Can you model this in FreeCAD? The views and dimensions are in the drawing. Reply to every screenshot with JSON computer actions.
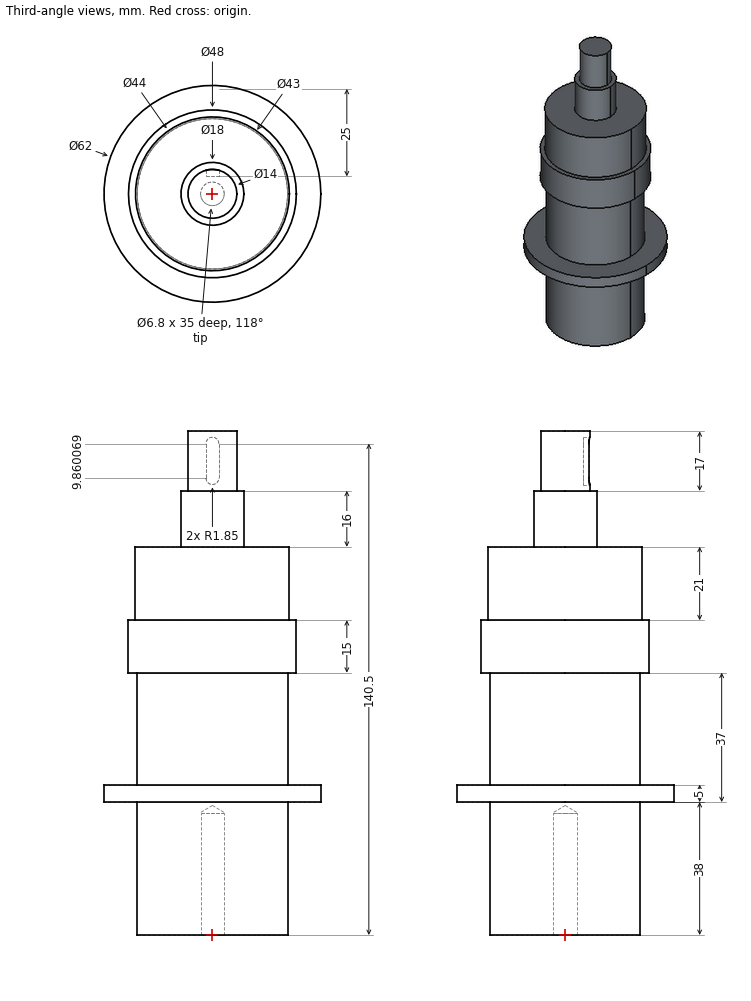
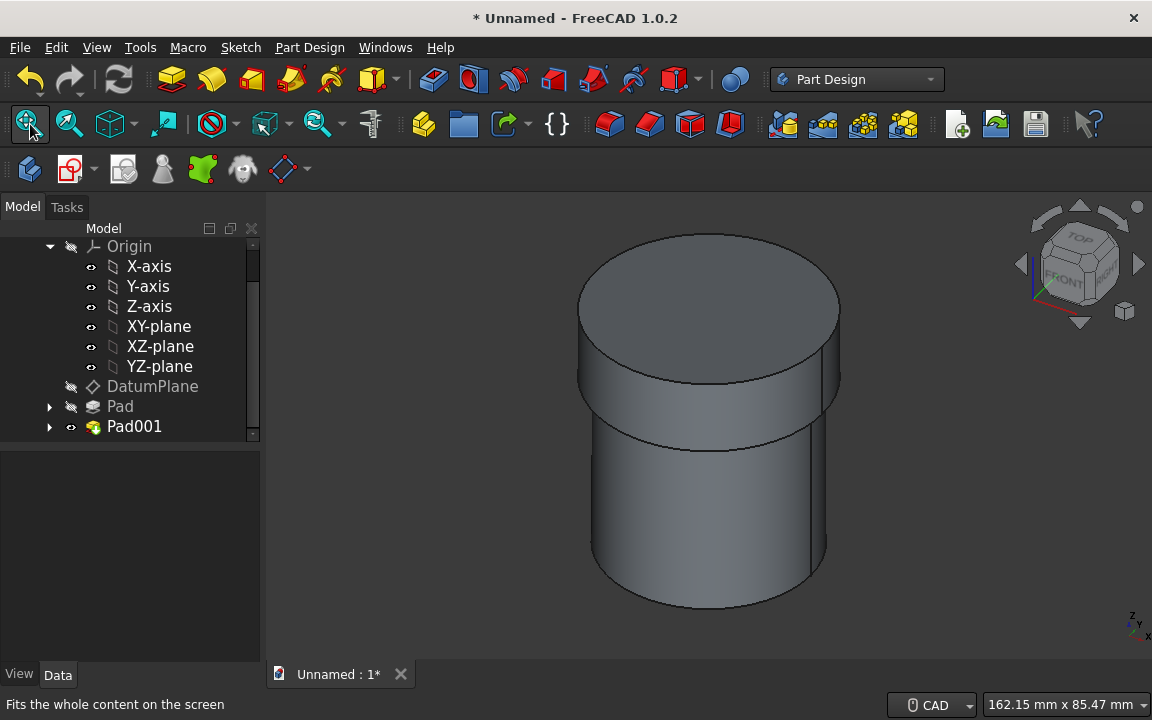
{"action": "left_click", "coordinate": [709, 308]}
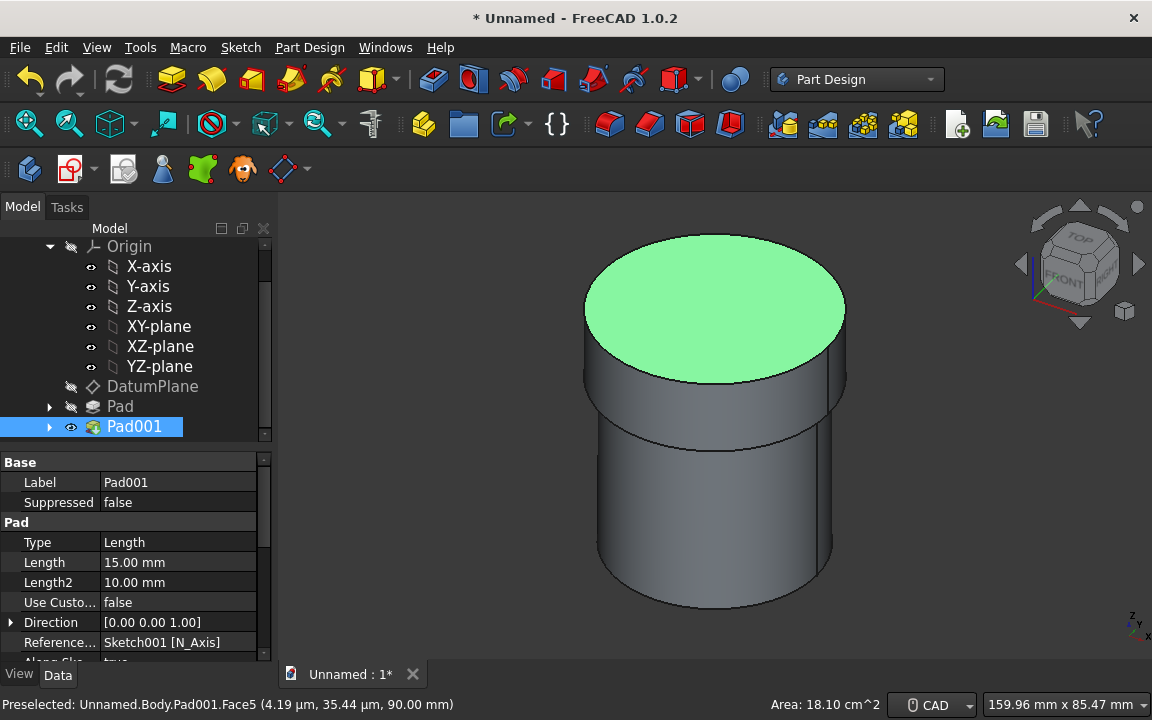
{"action": "left_click", "coordinate": [70, 170]}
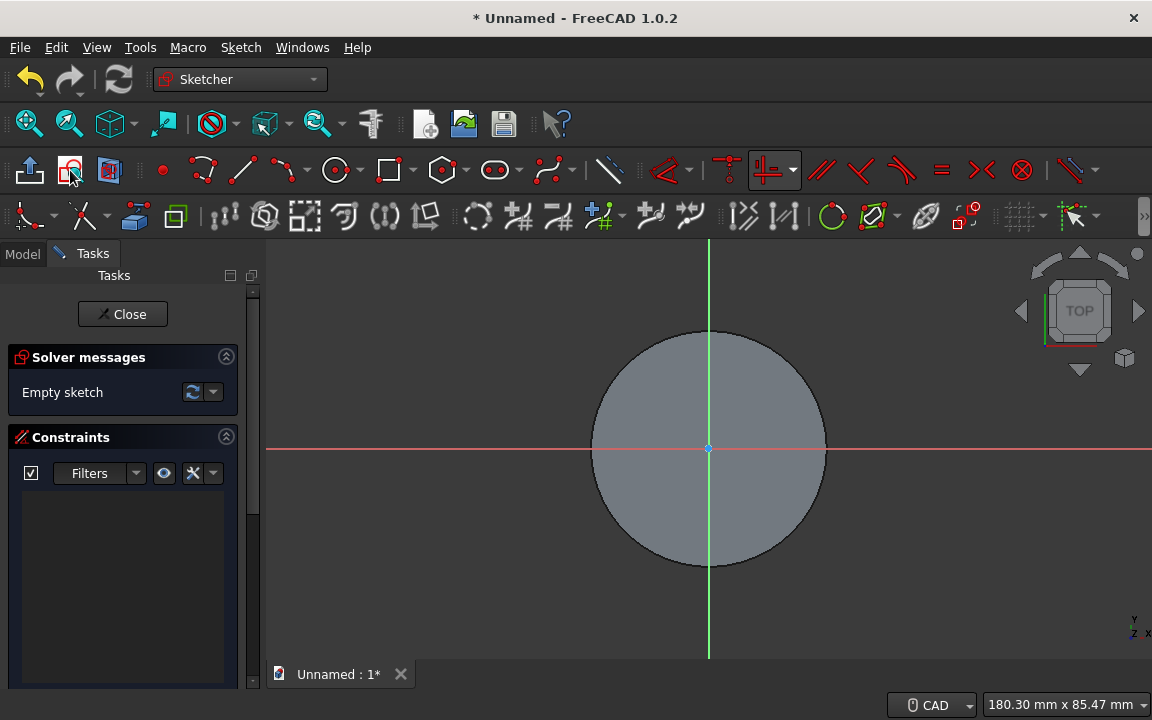
{"action": "left_click", "coordinate": [336, 170]}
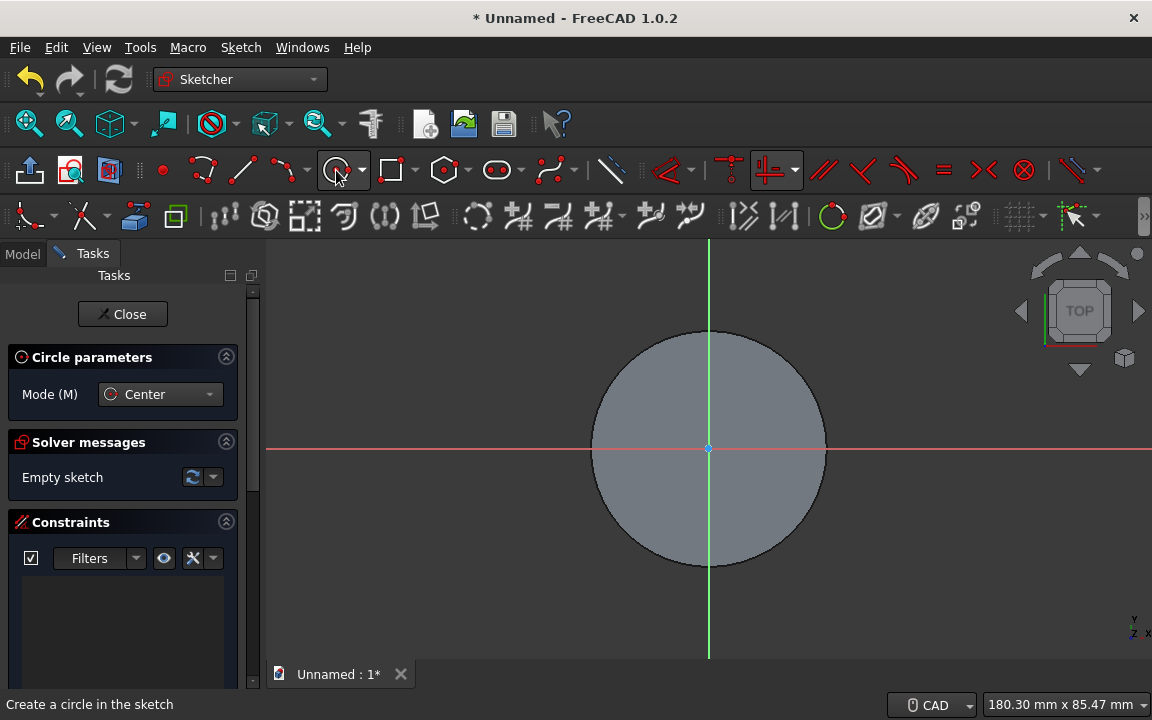
{"action": "left_click", "coordinate": [709, 449]}
{"action": "left_click", "coordinate": [785, 373]}
{"action": "key", "text": "Escape"}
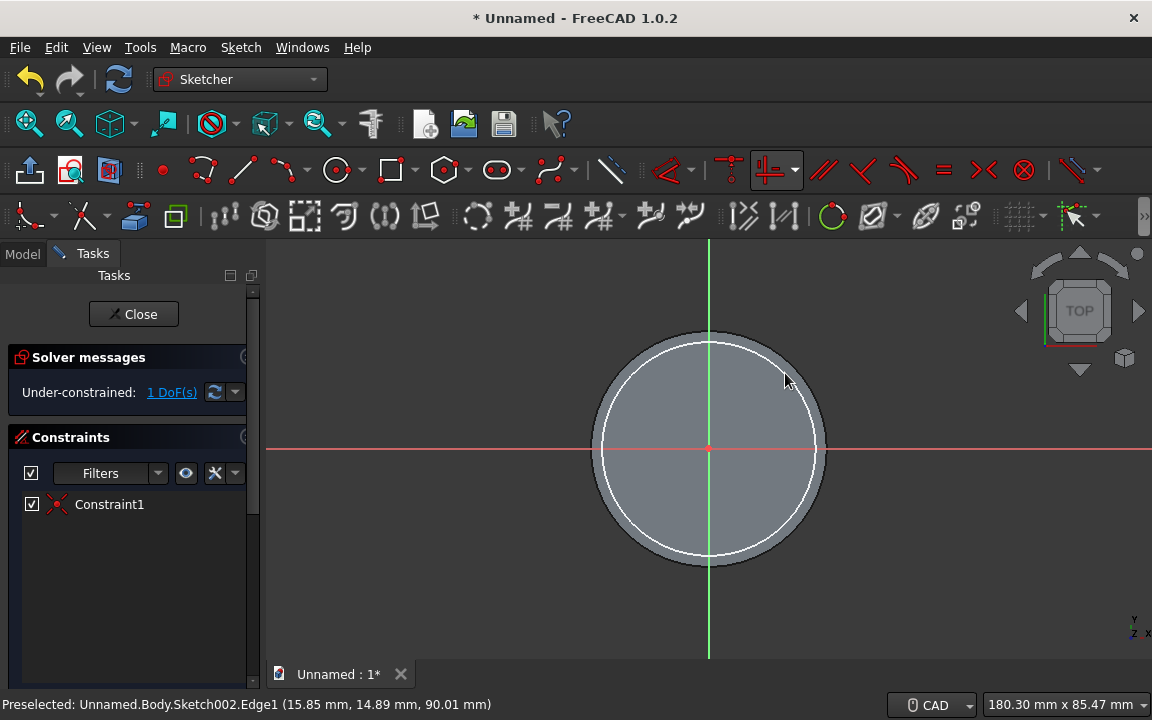
{"action": "left_click", "coordinate": [666, 170]}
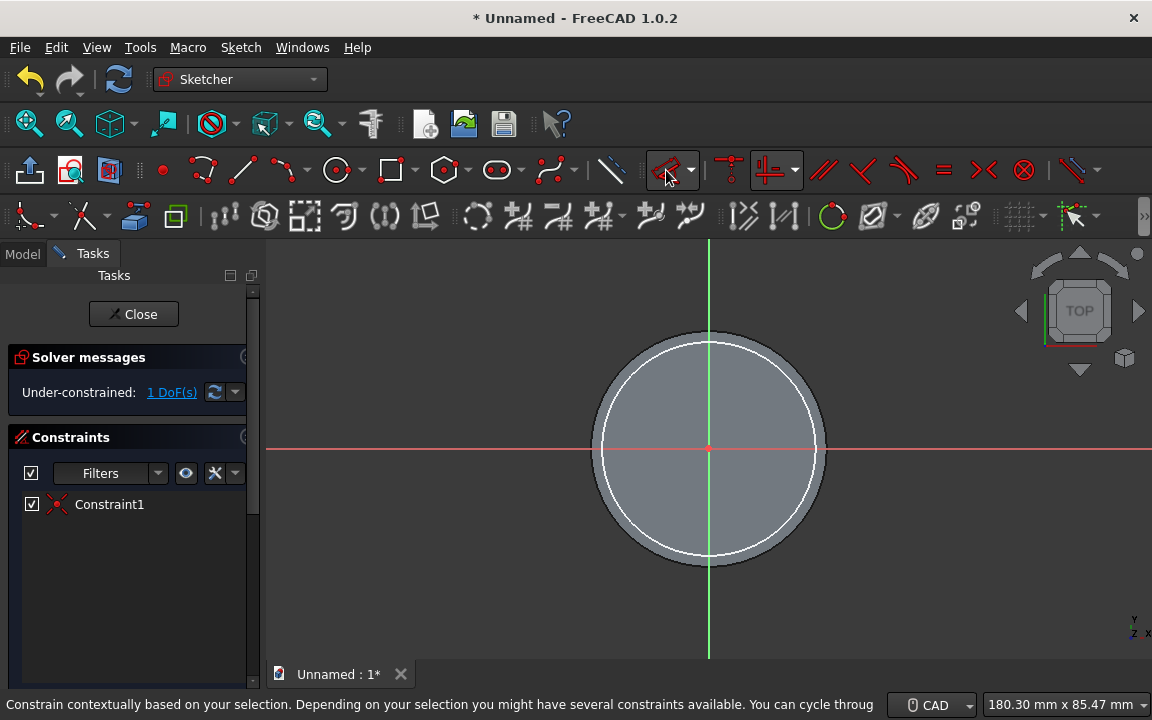
{"action": "left_click", "coordinate": [784, 373]}
{"action": "left_click", "coordinate": [806, 350]}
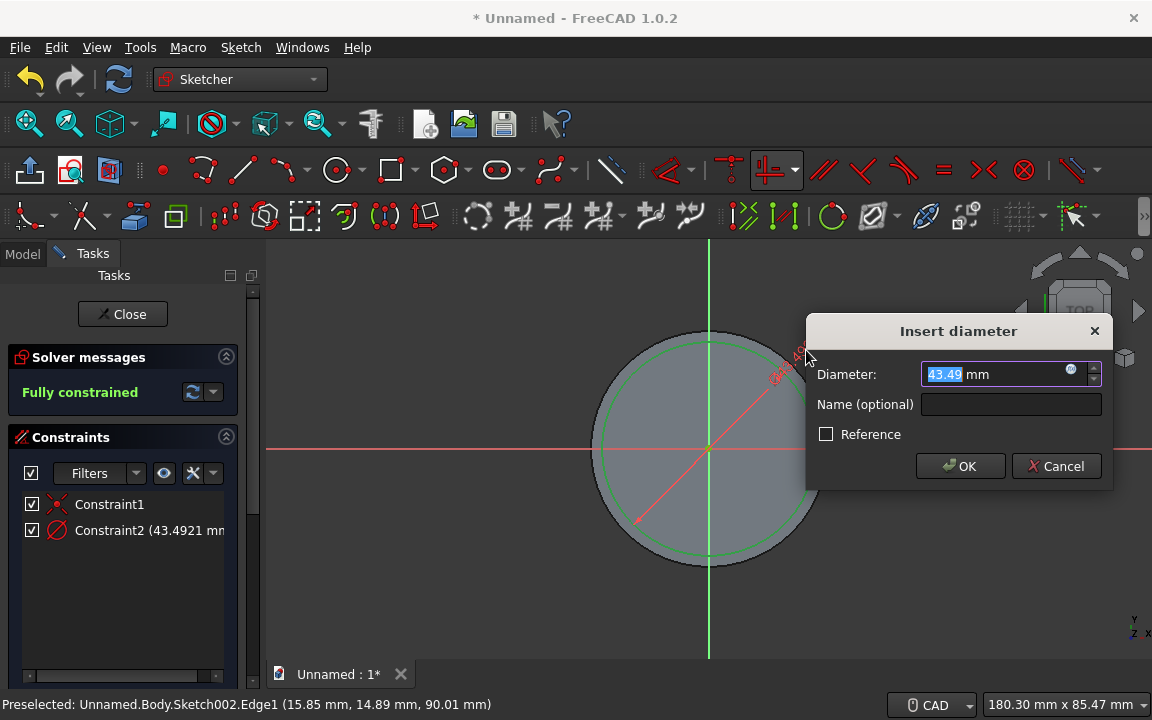
{"action": "type", "text": "44"}
{"action": "key", "text": "Return"}
{"action": "key", "text": "Escape"}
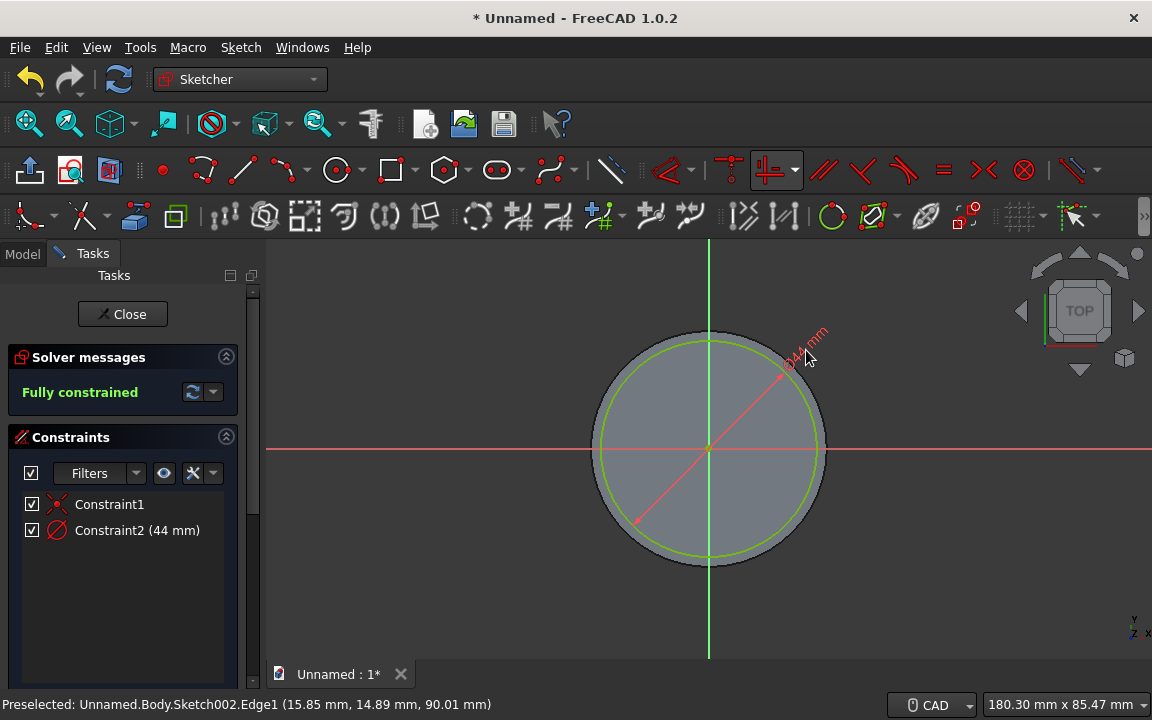
{"action": "left_click", "coordinate": [123, 314]}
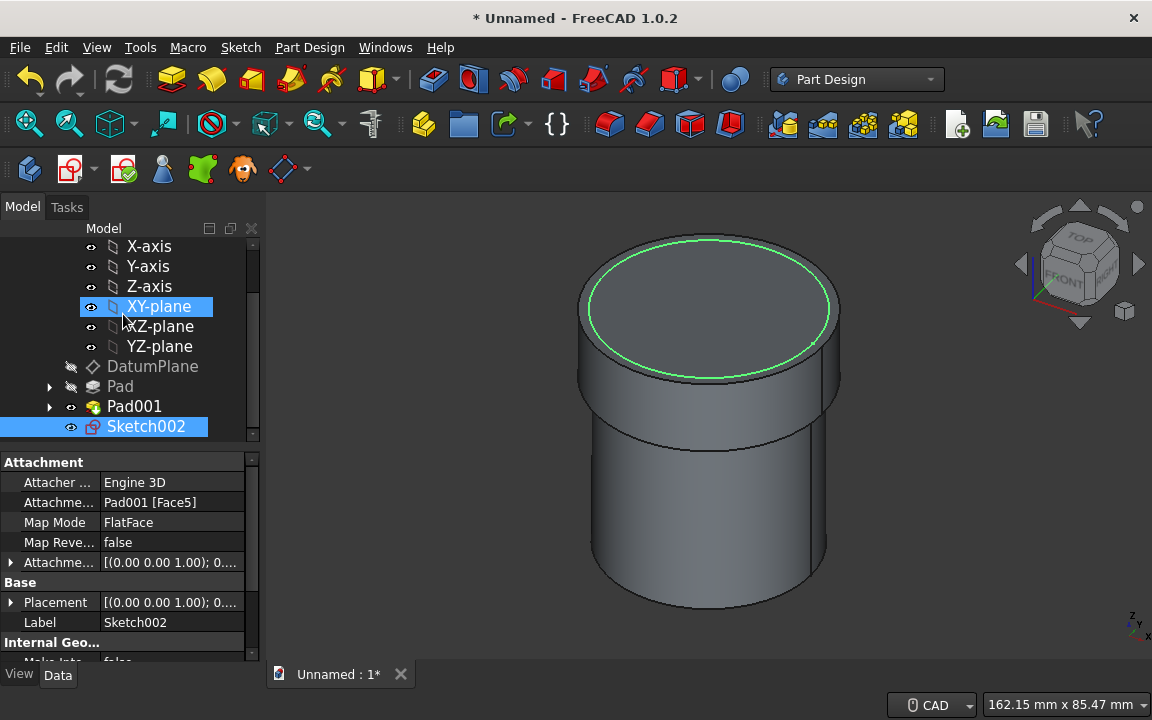
{"action": "left_click", "coordinate": [172, 80]}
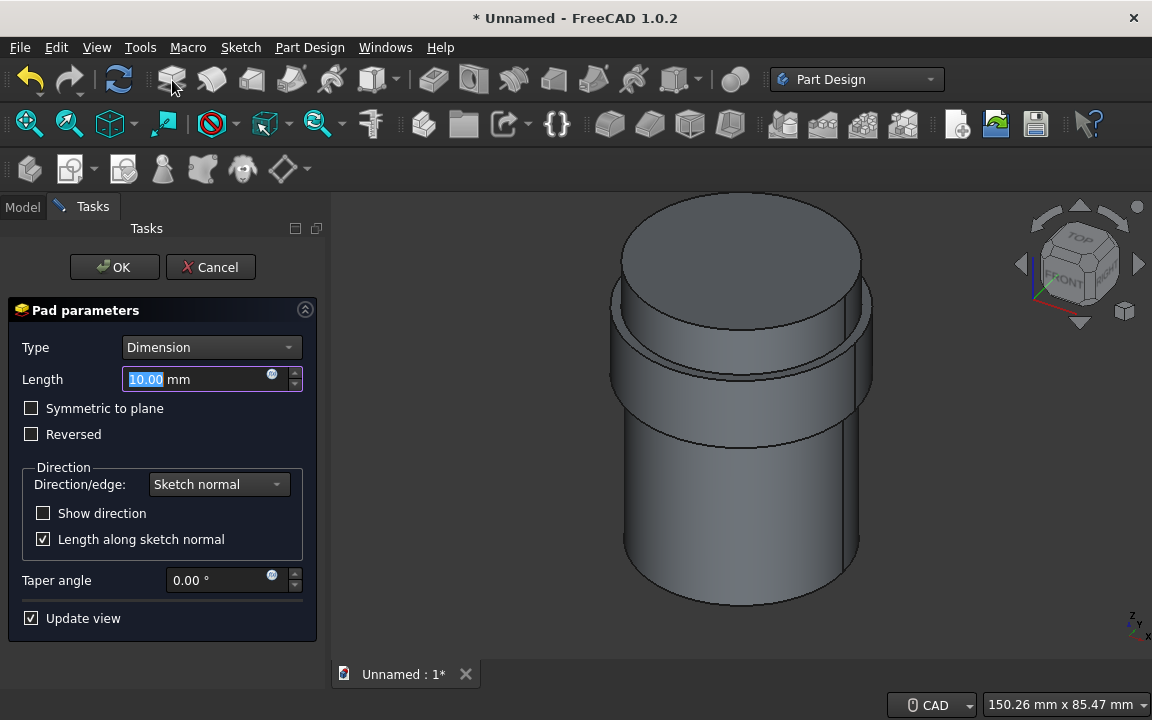
{"action": "type", "text": "21"}
{"action": "key", "text": "Tab"}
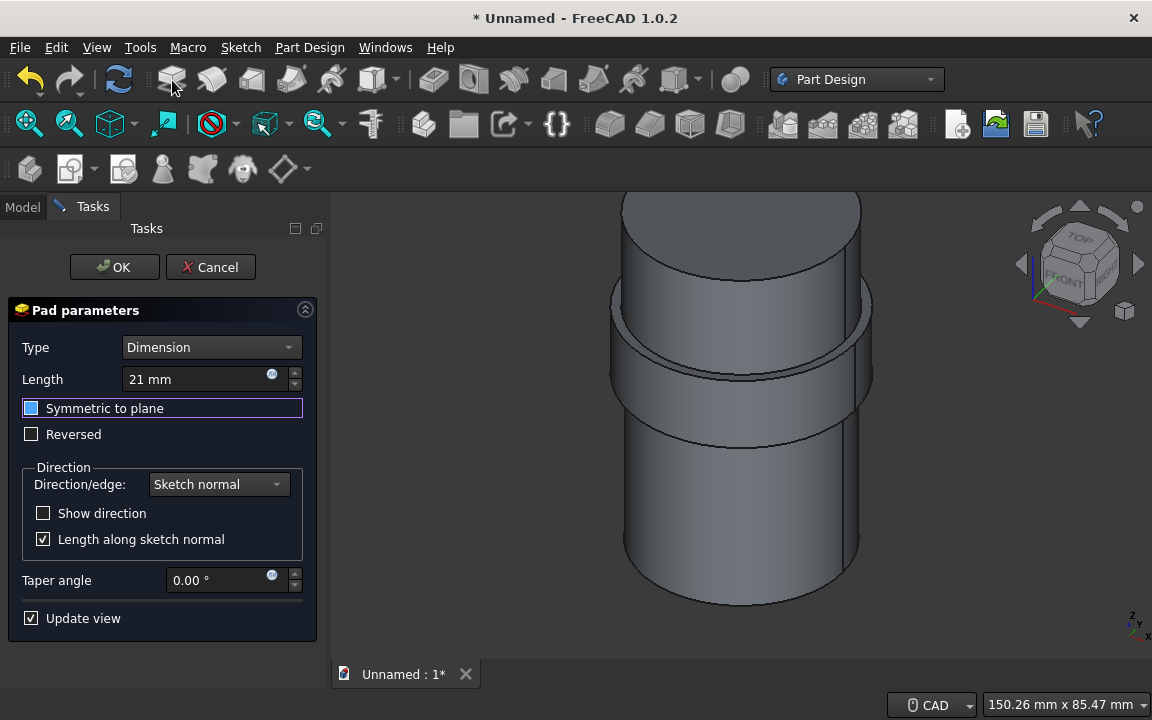
{"action": "left_click", "coordinate": [115, 267]}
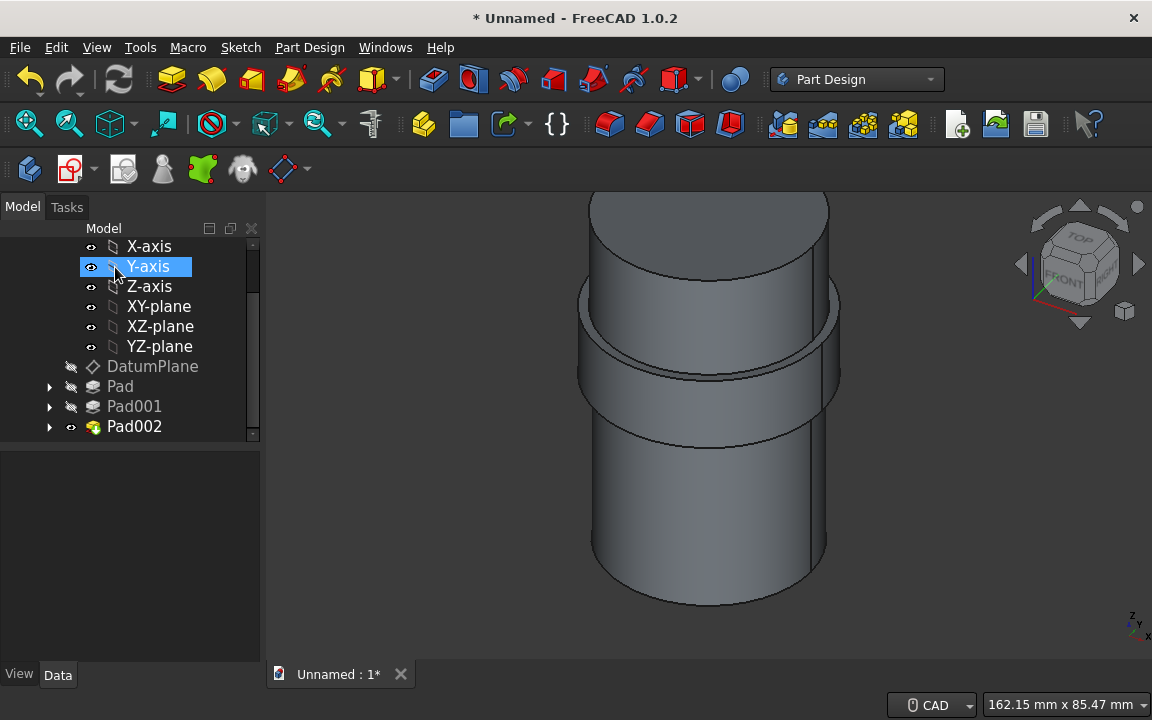
{"action": "left_click", "coordinate": [30, 124]}